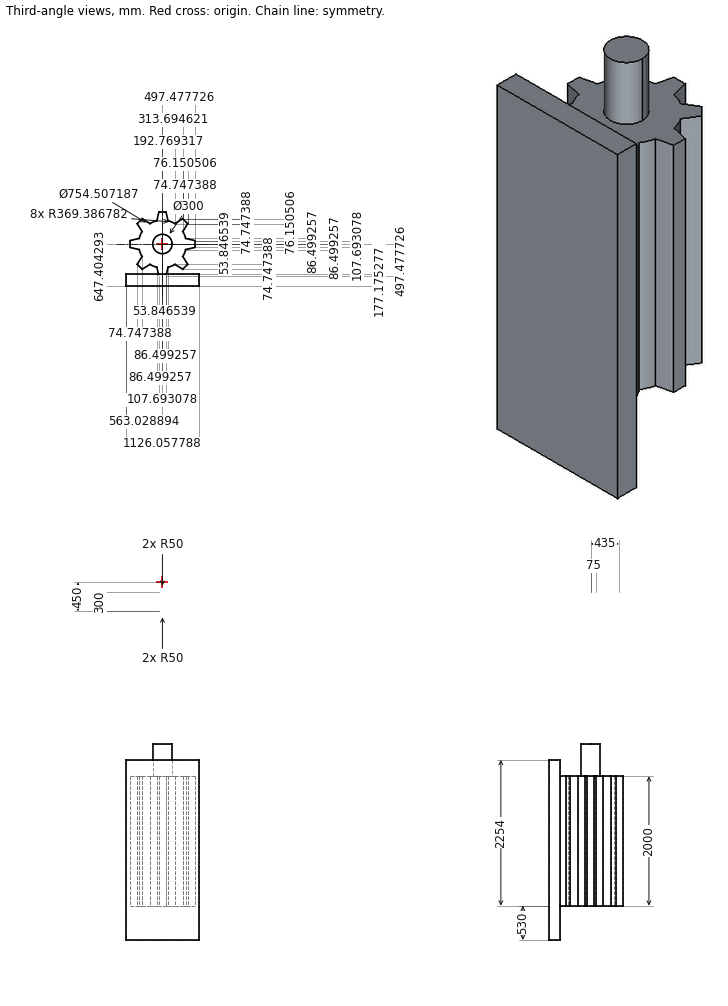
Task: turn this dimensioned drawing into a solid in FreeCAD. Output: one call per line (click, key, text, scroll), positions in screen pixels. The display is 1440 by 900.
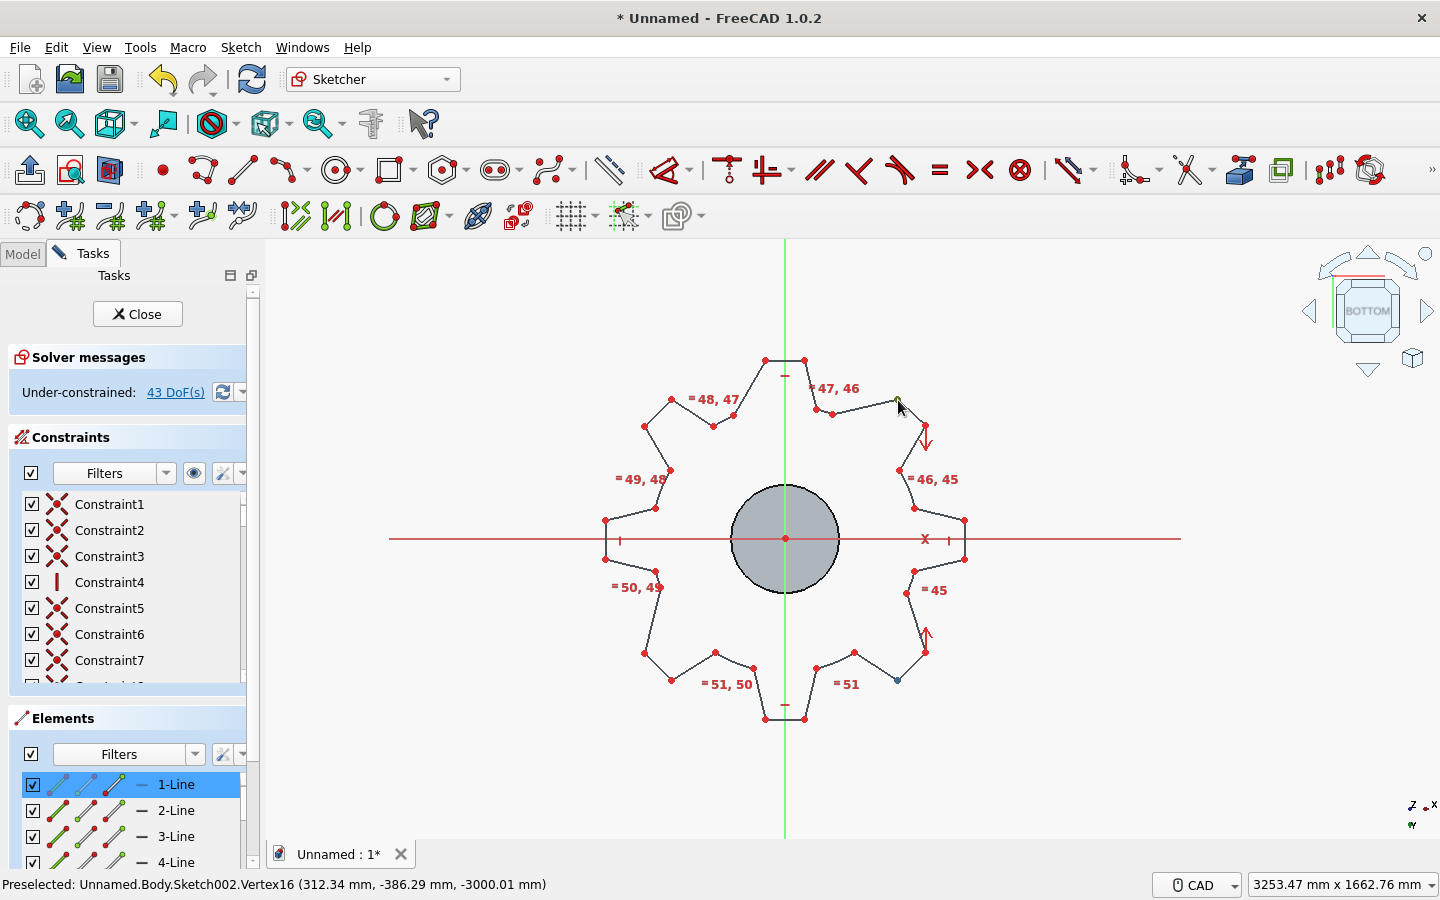
click(434, 539)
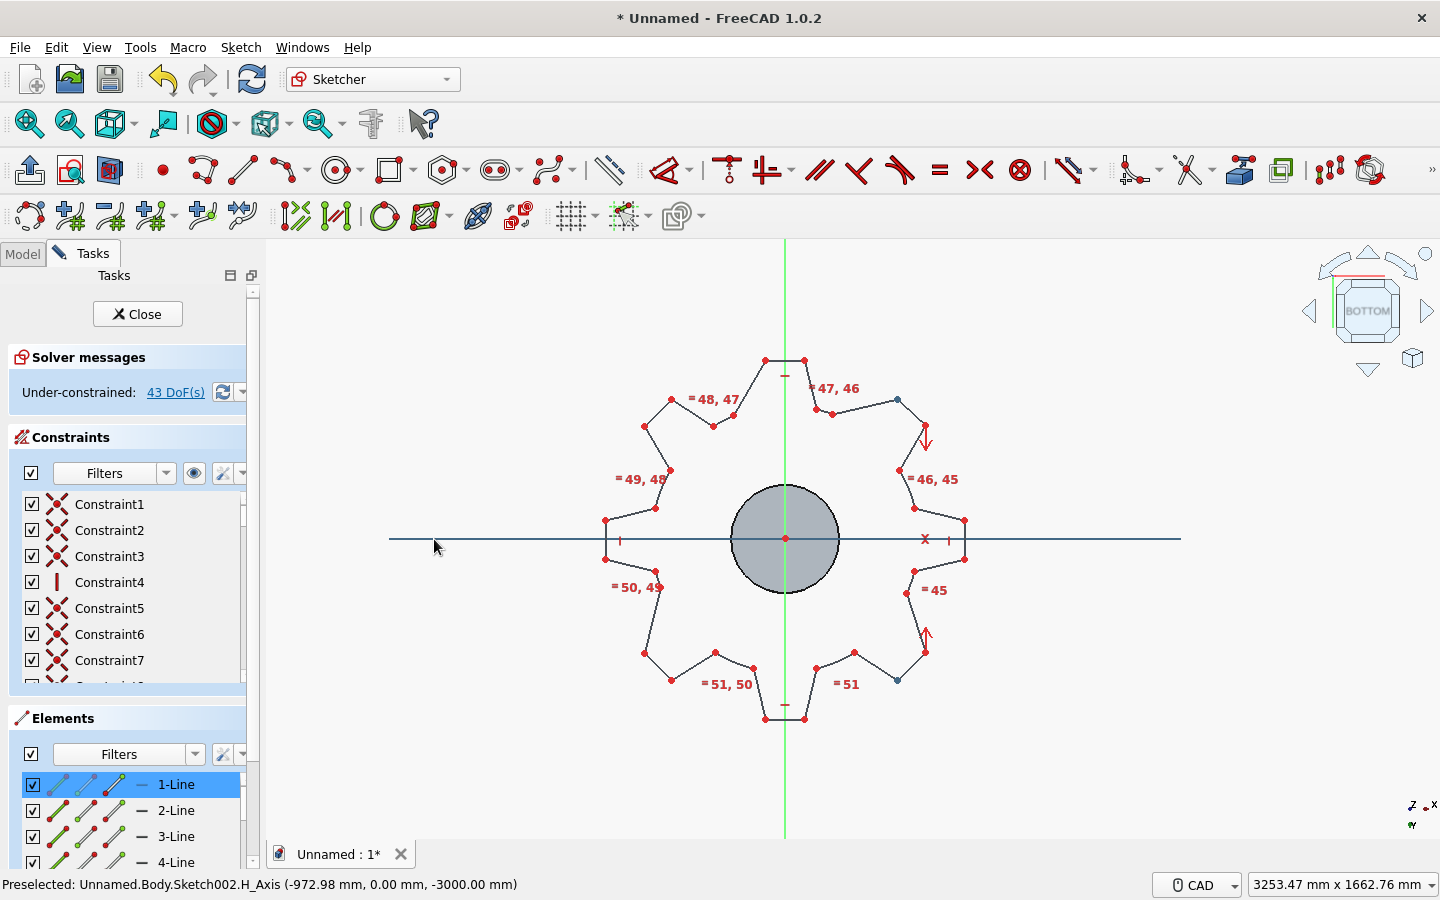
click(980, 170)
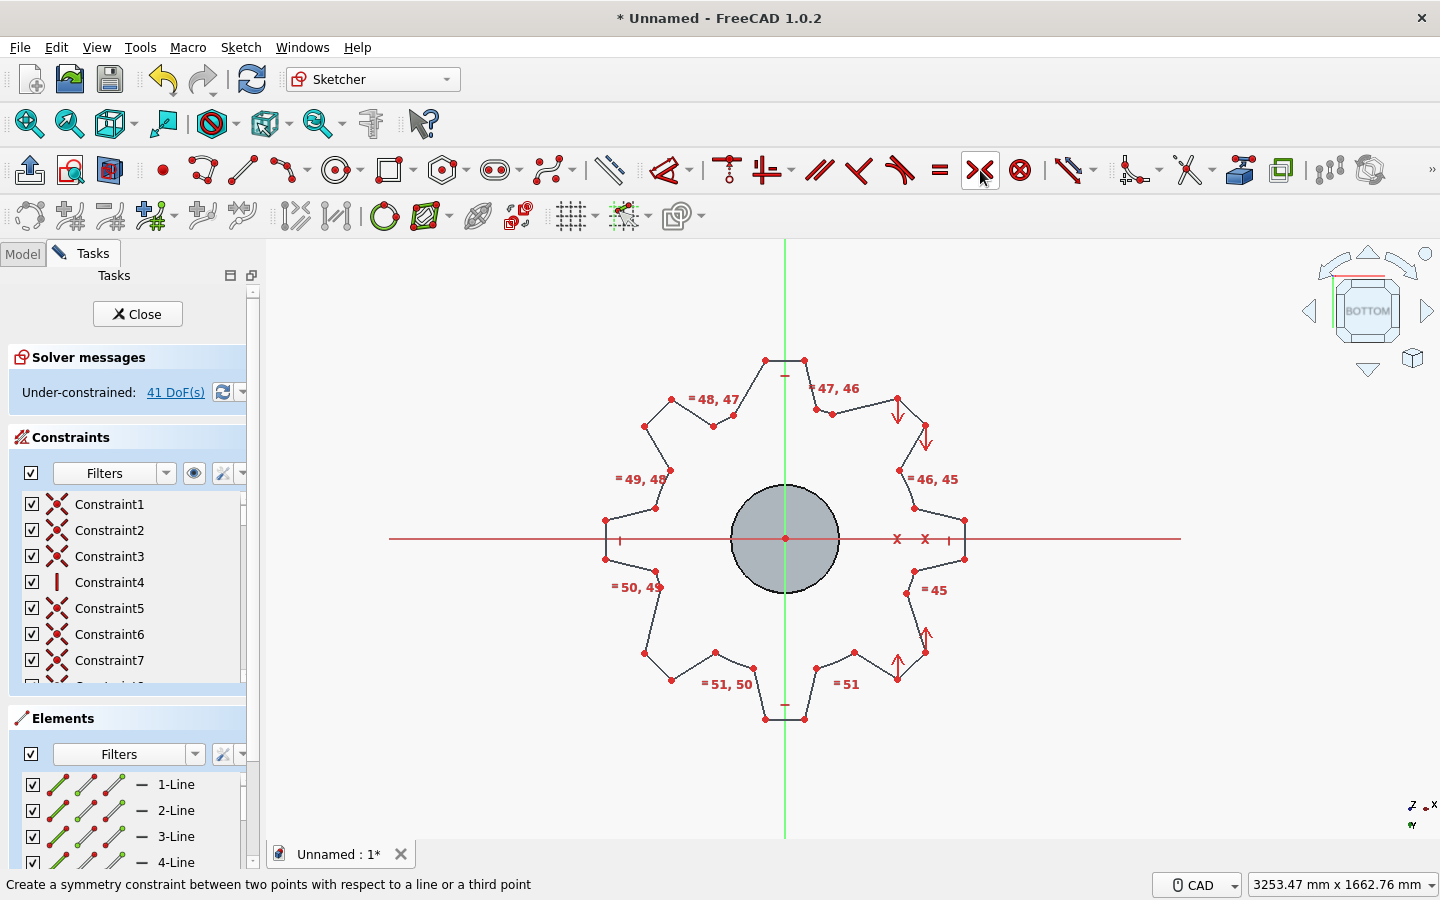
click(898, 399)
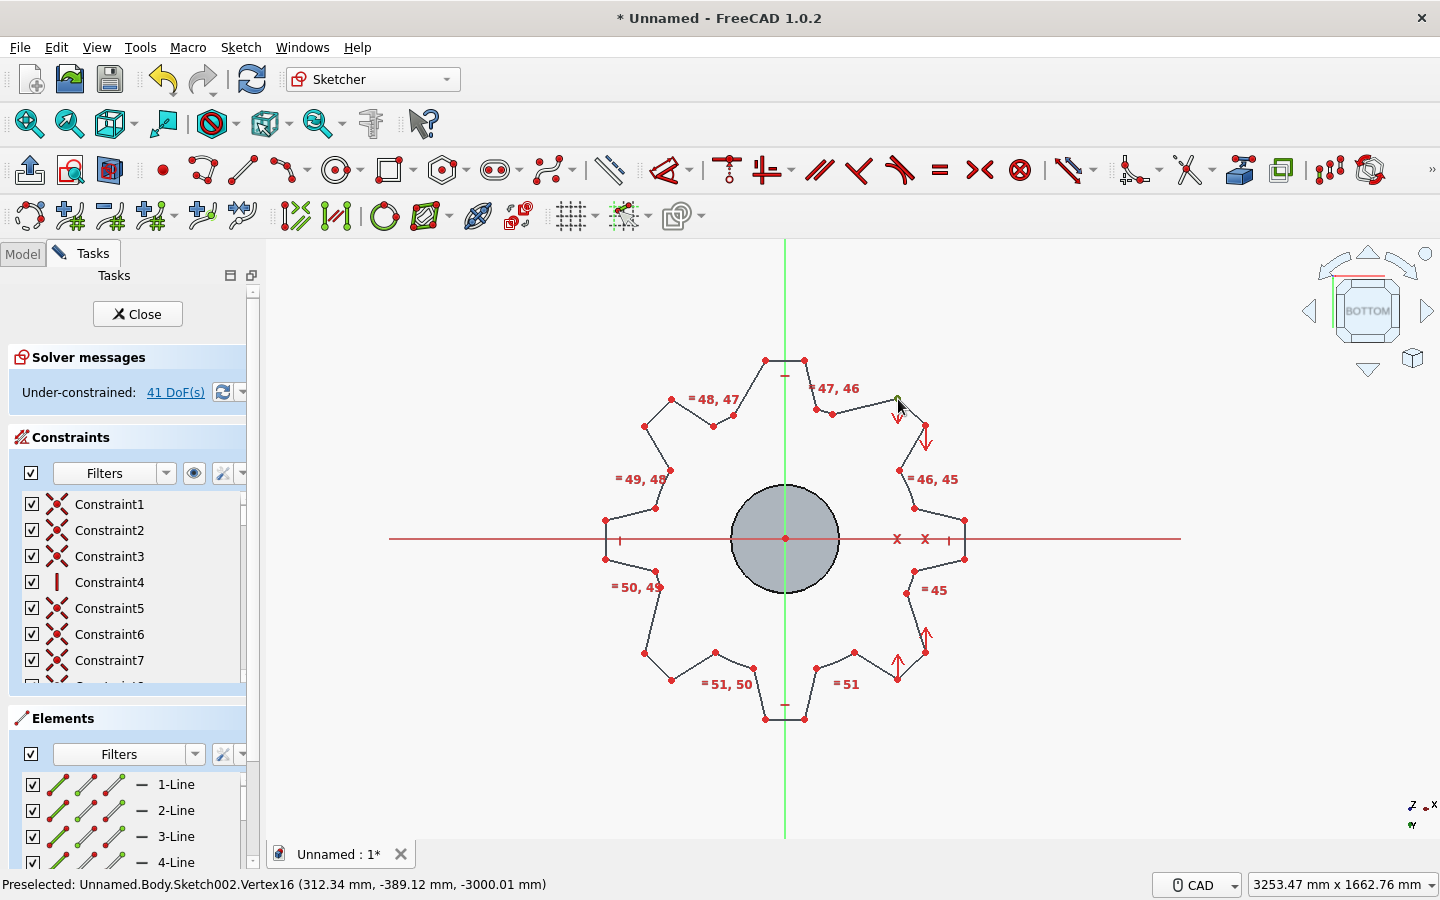
click(672, 400)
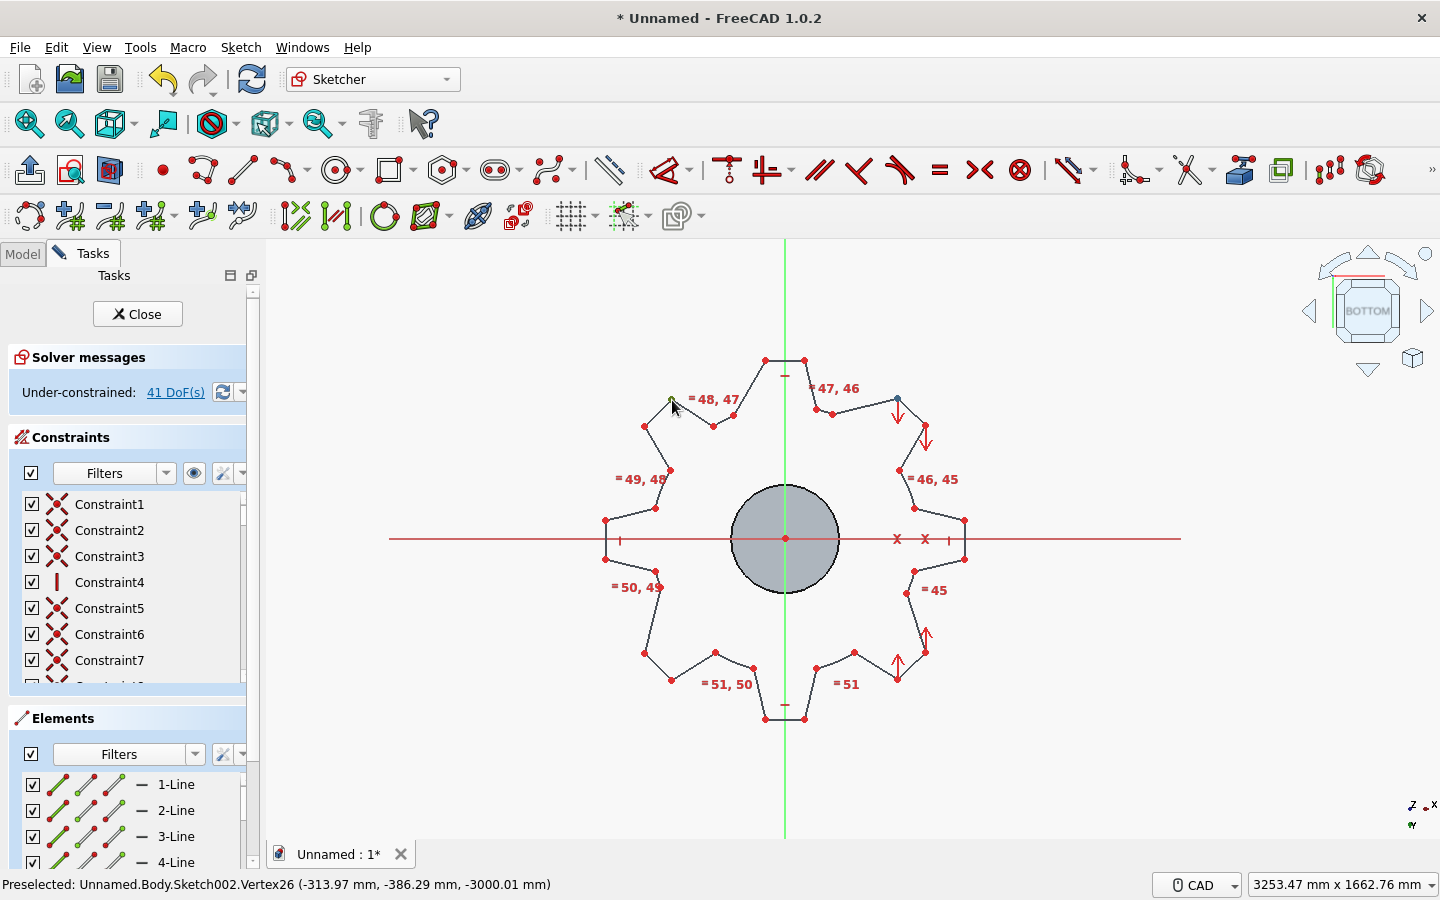
click(785, 772)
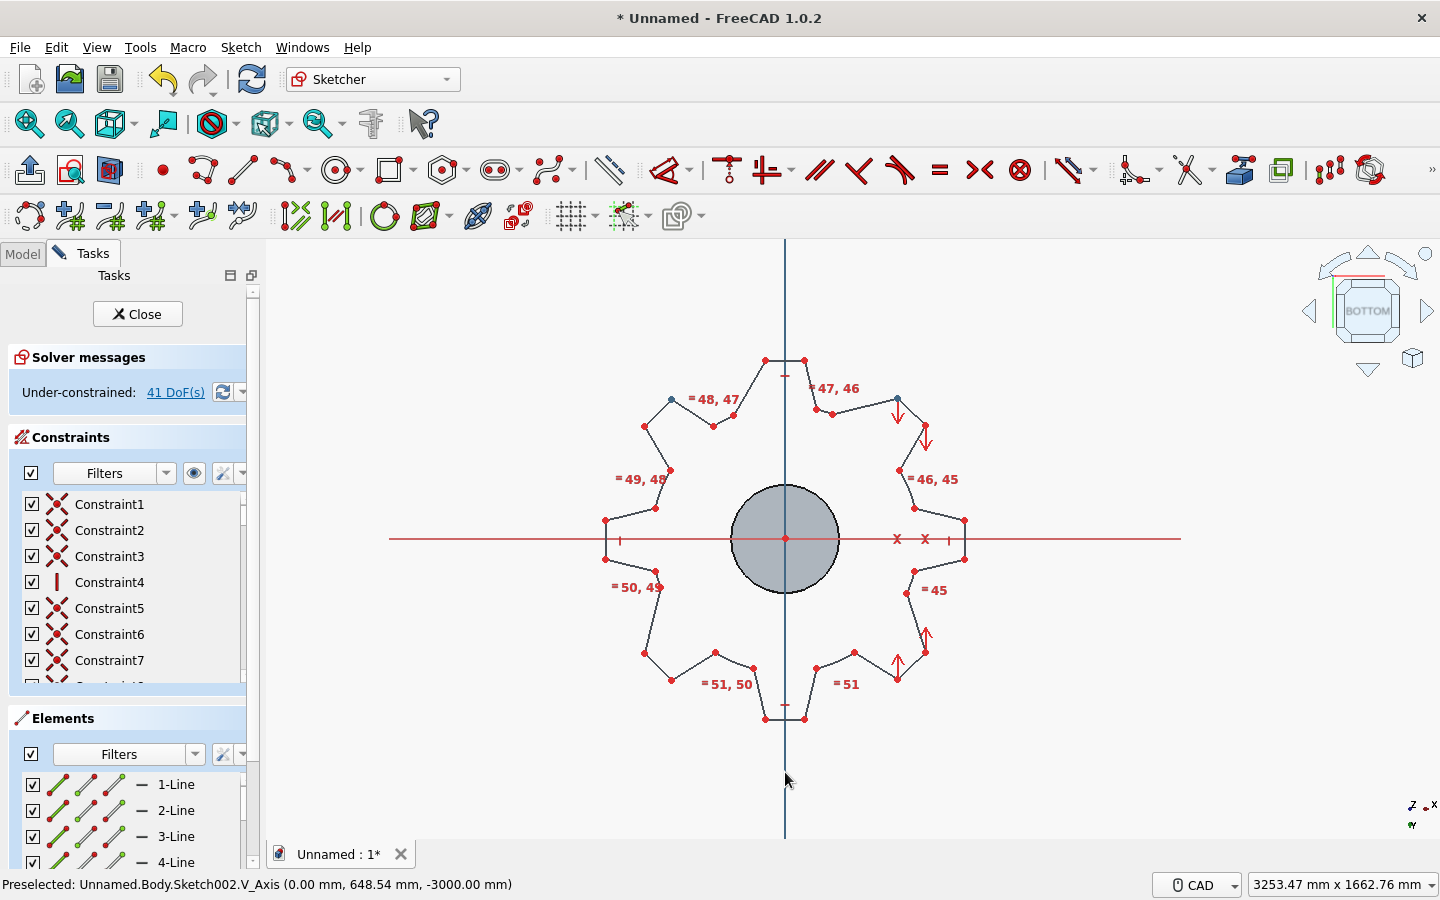
click(980, 170)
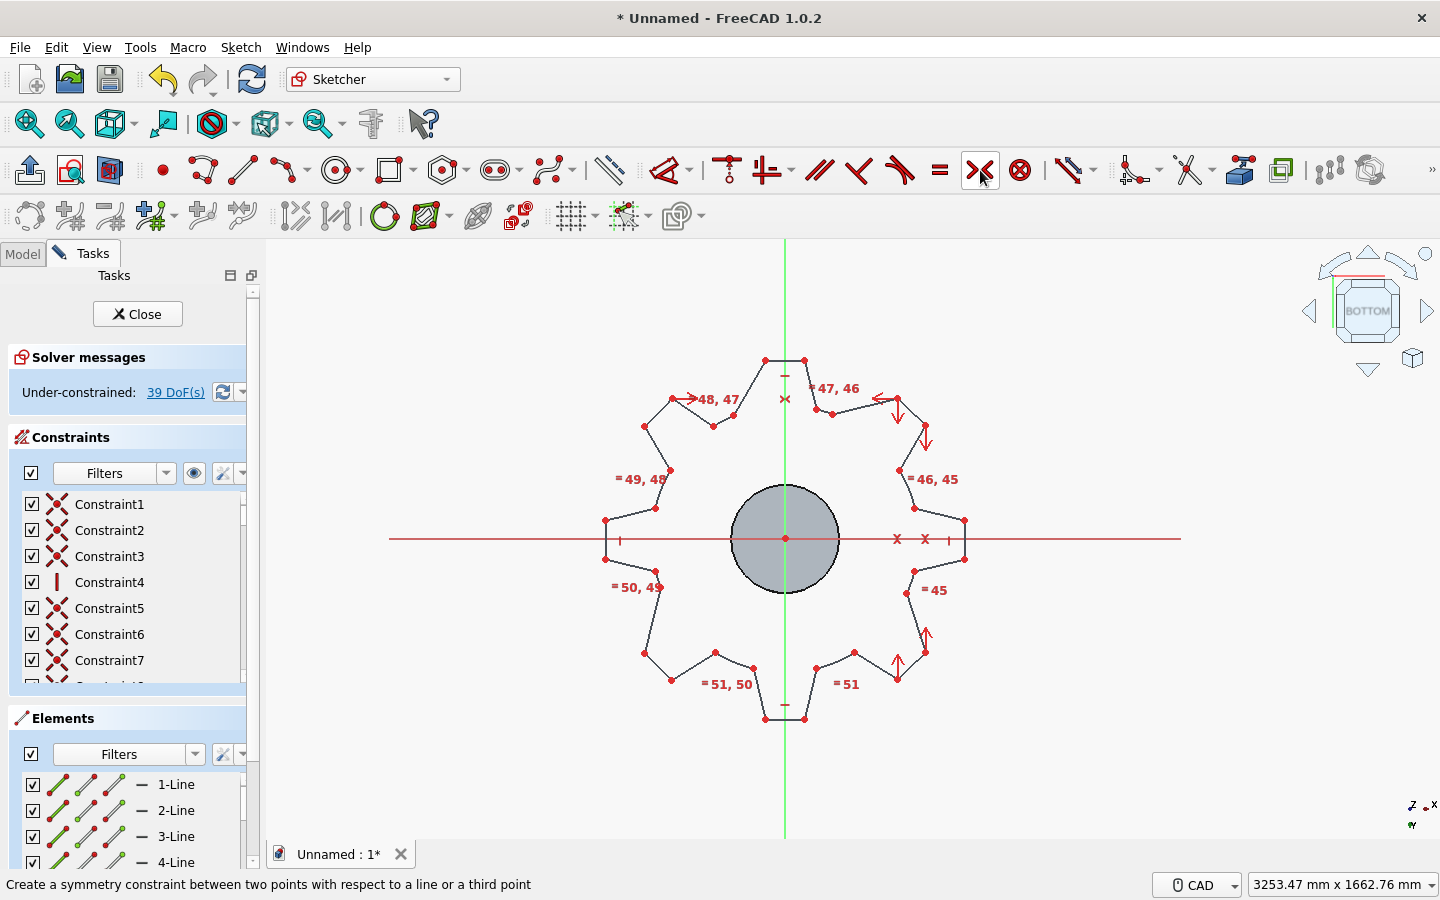
click(926, 425)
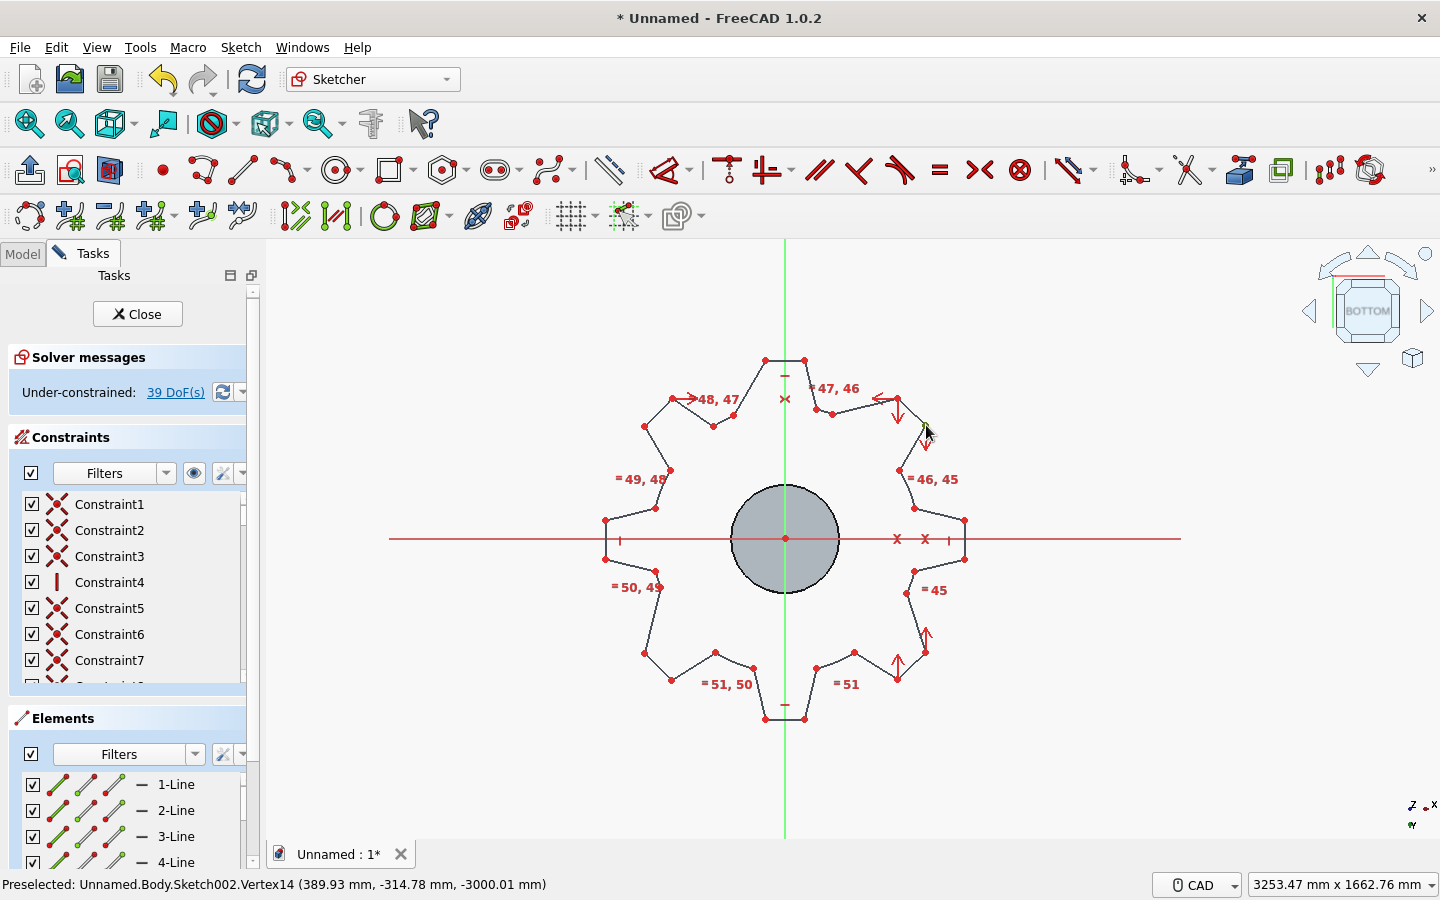
click(645, 427)